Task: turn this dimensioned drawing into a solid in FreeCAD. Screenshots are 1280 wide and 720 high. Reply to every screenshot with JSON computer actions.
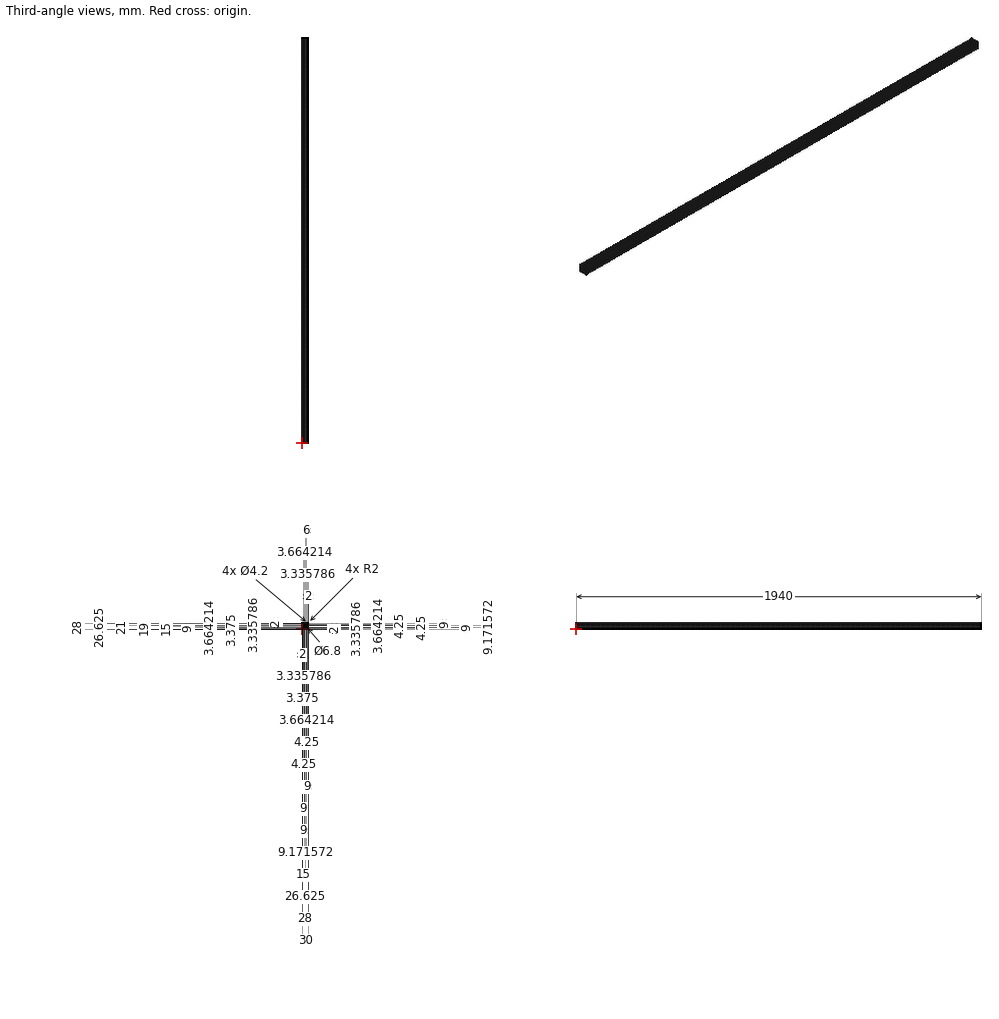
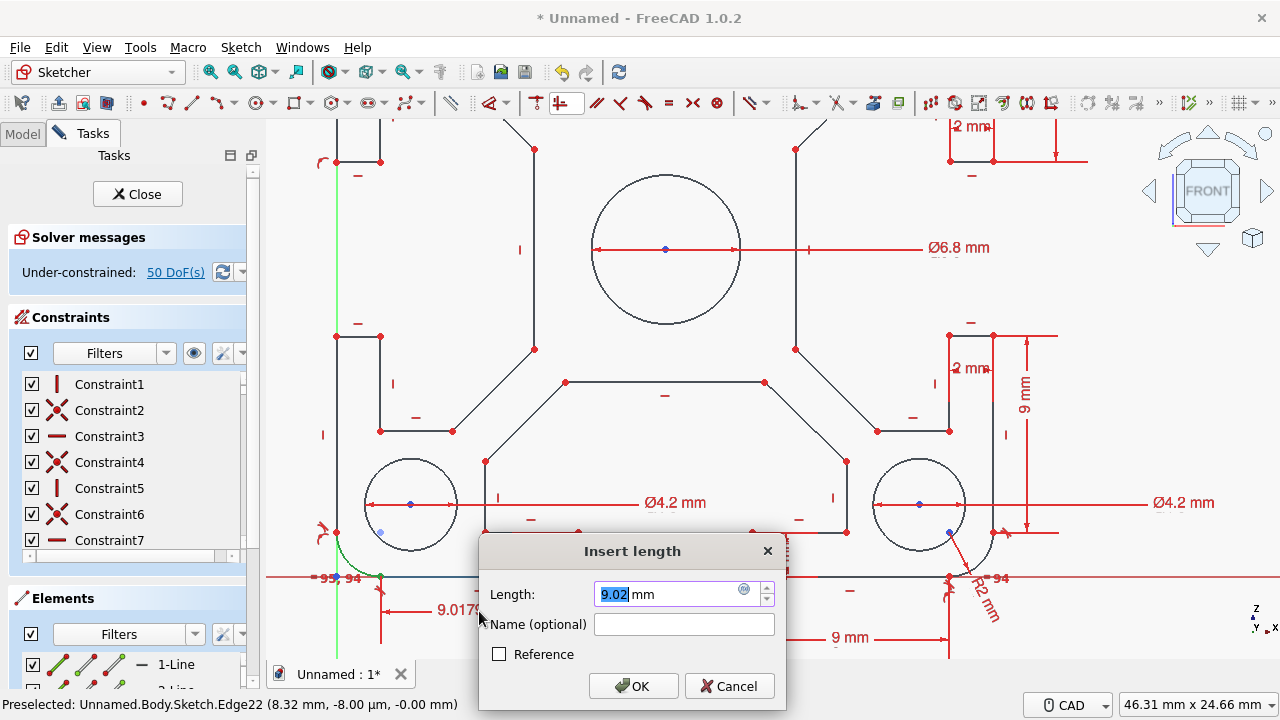
{"action": "type", "text": "9"}
{"action": "key", "text": "Return"}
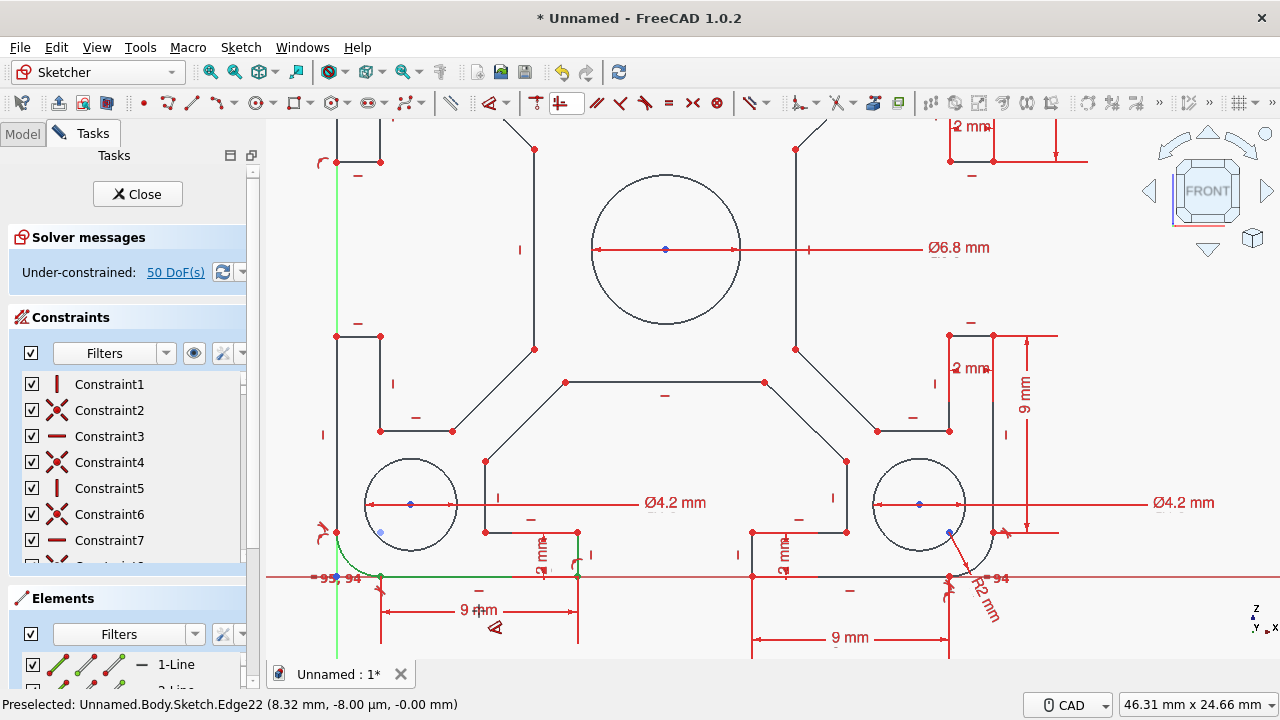
{"action": "left_click", "coordinate": [337, 474]}
{"action": "left_click", "coordinate": [303, 435]}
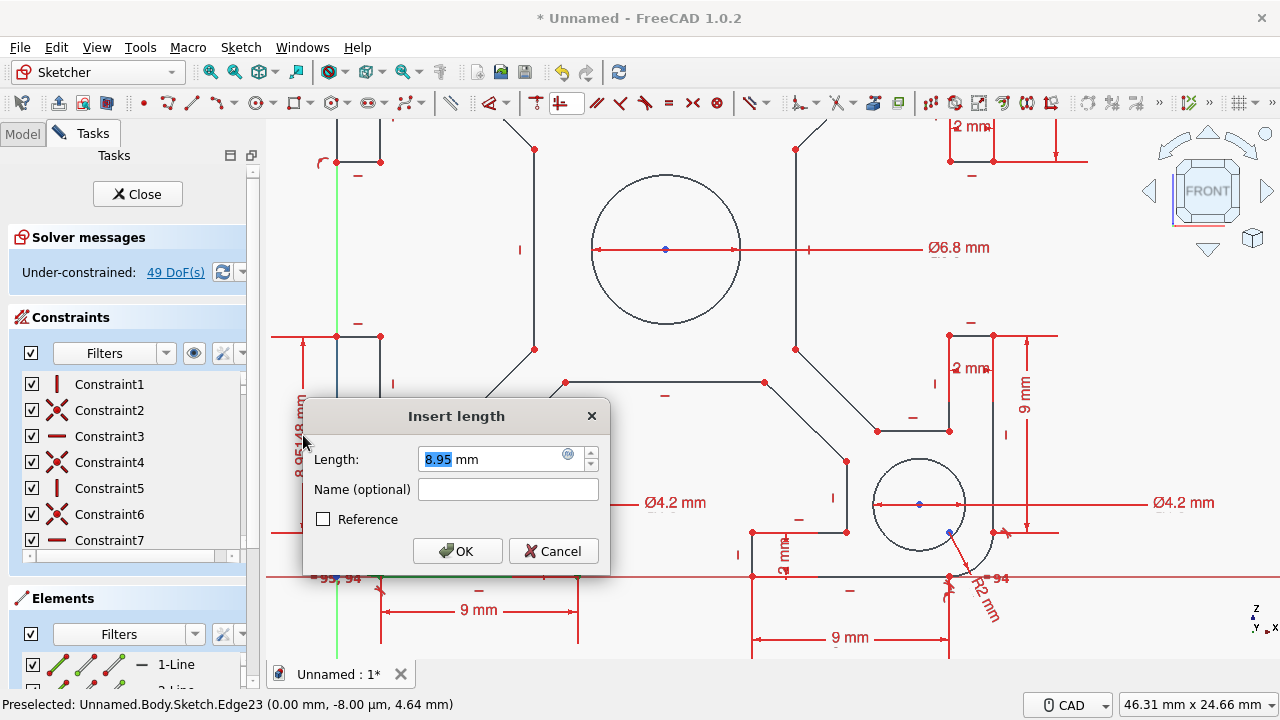
{"action": "type", "text": "9"}
{"action": "key", "text": "Return"}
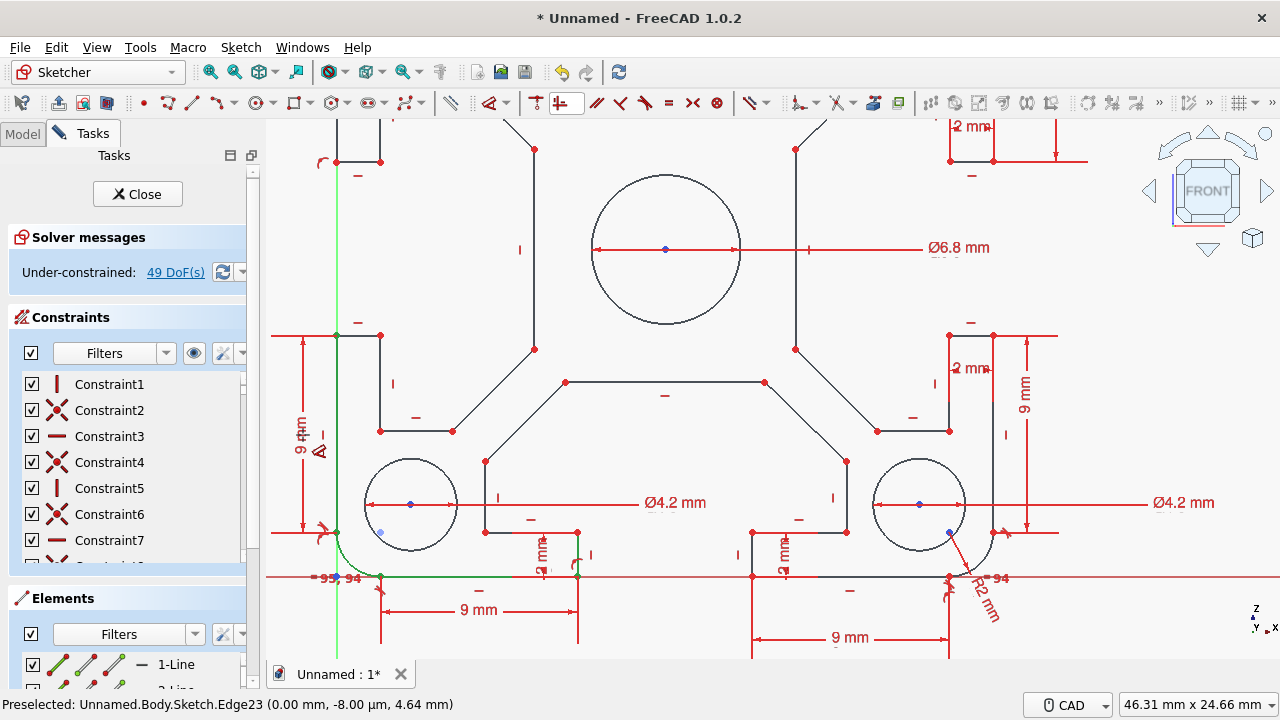
{"action": "left_click", "coordinate": [350, 336]}
{"action": "left_click", "coordinate": [358, 370]}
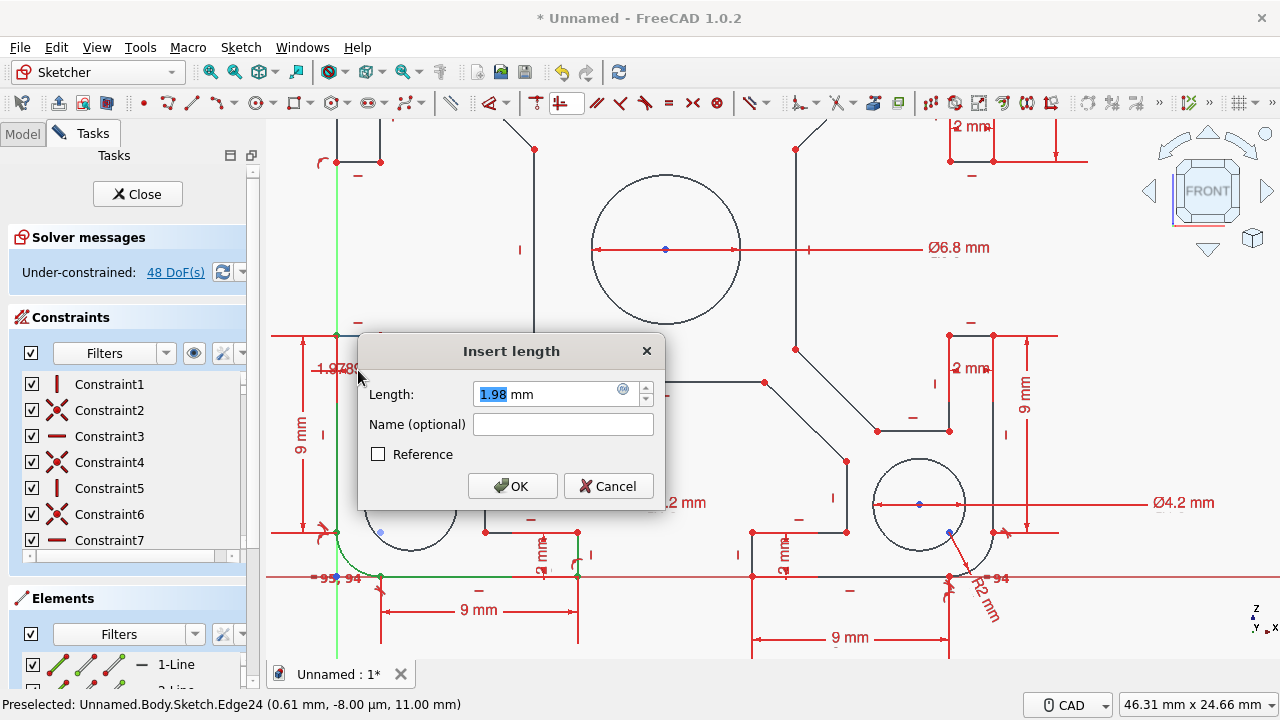
{"action": "type", "text": "2"}
{"action": "key", "text": "Return"}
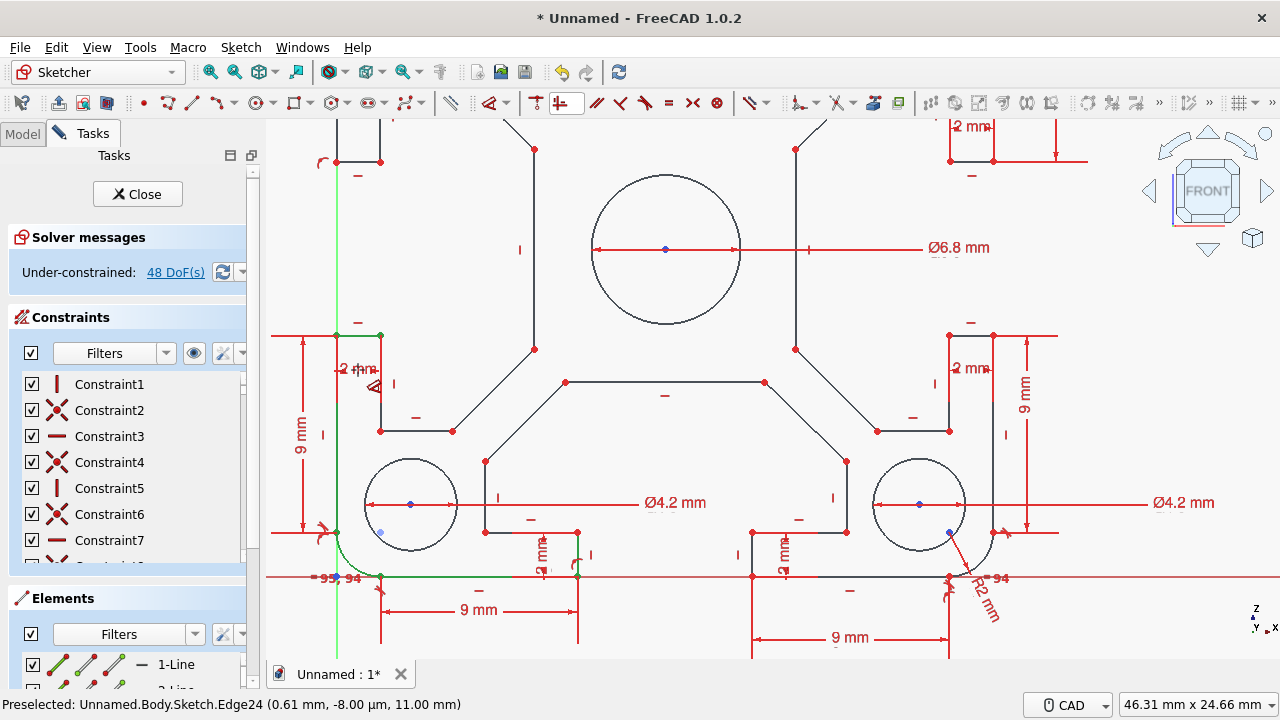
{"action": "left_click", "coordinate": [367, 162]}
{"action": "left_click", "coordinate": [358, 196]}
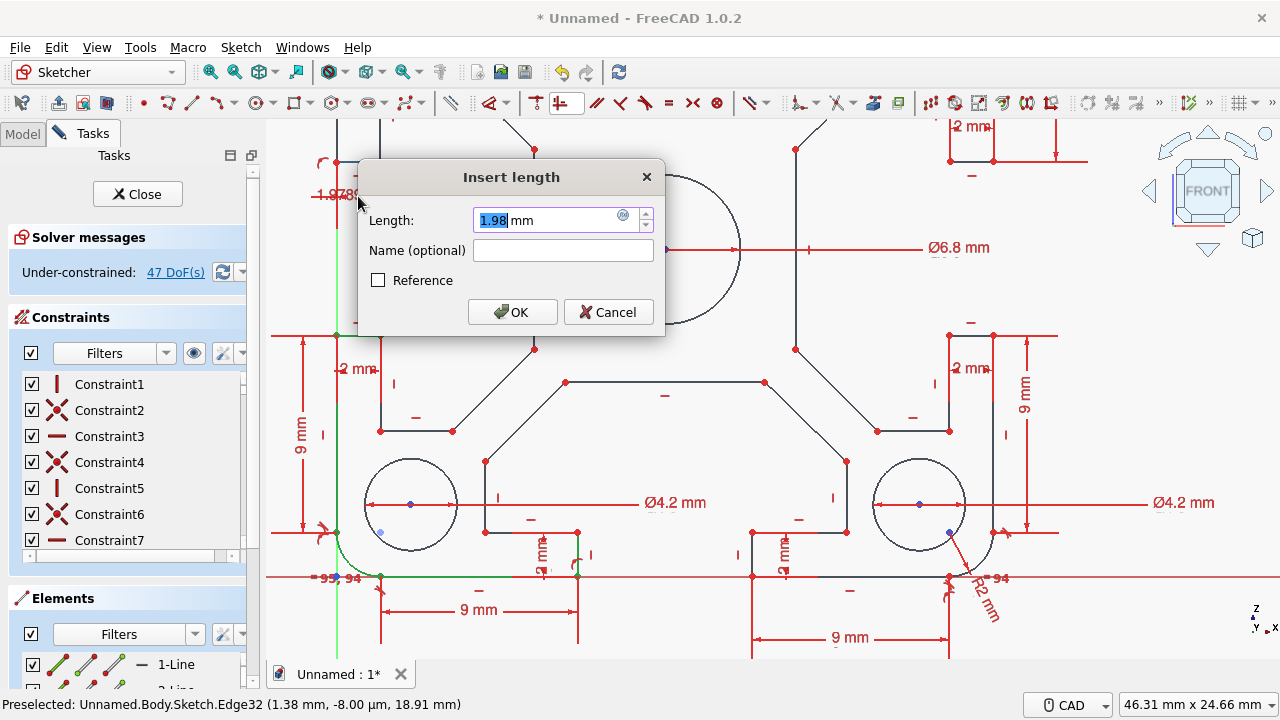
{"action": "type", "text": "2"}
{"action": "key", "text": "Return"}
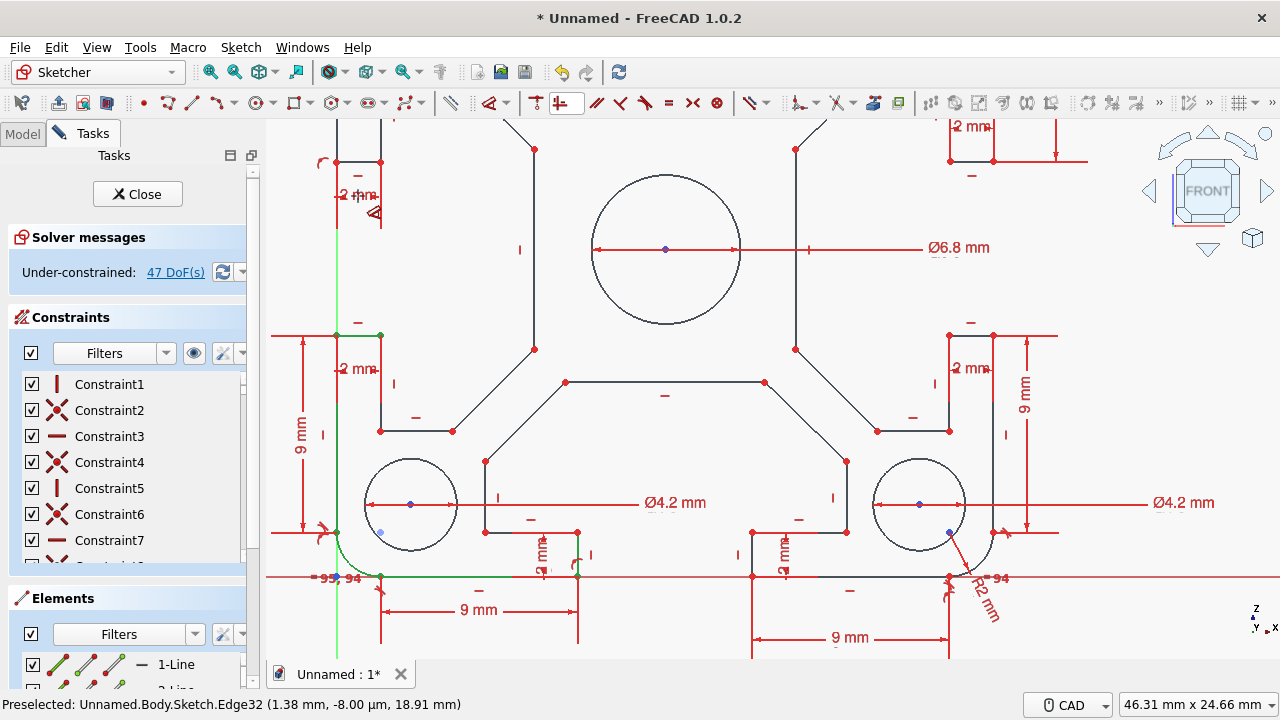
{"action": "scroll", "coordinate": [752, 560], "scroll_direction": "down", "scroll_amount": 3}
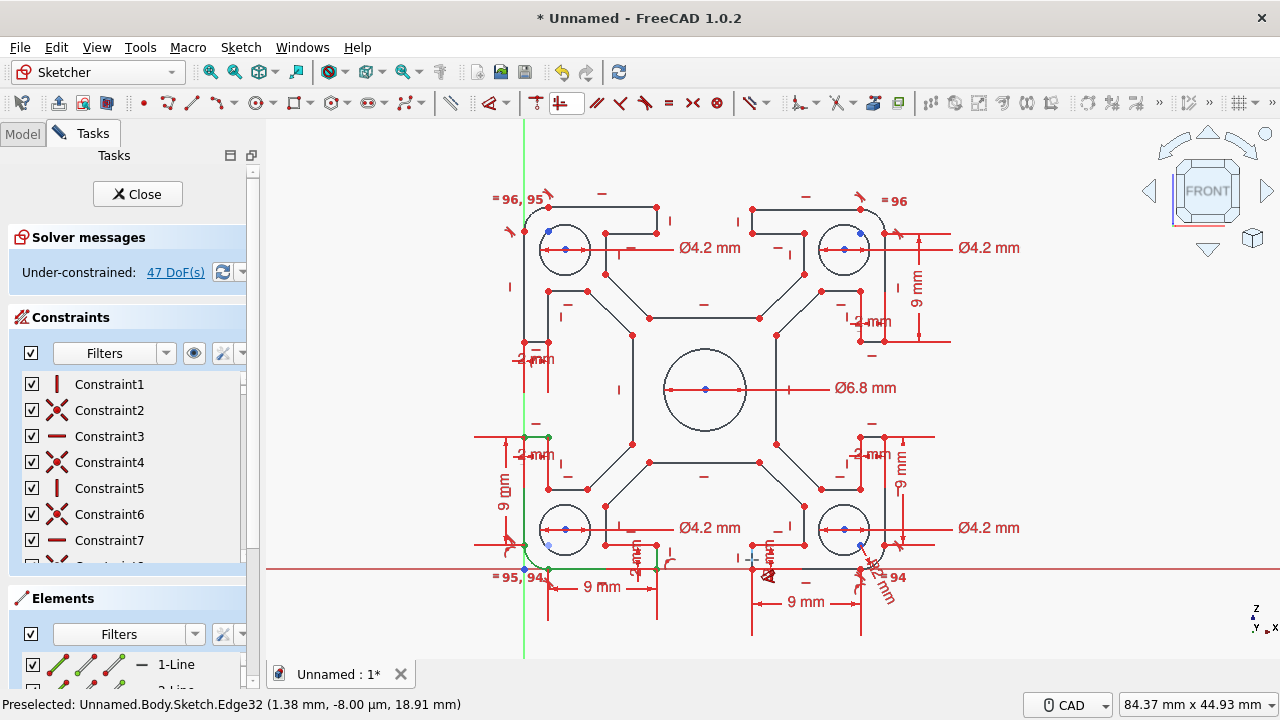
{"action": "left_click", "coordinate": [524, 309]}
{"action": "left_click", "coordinate": [490, 287]}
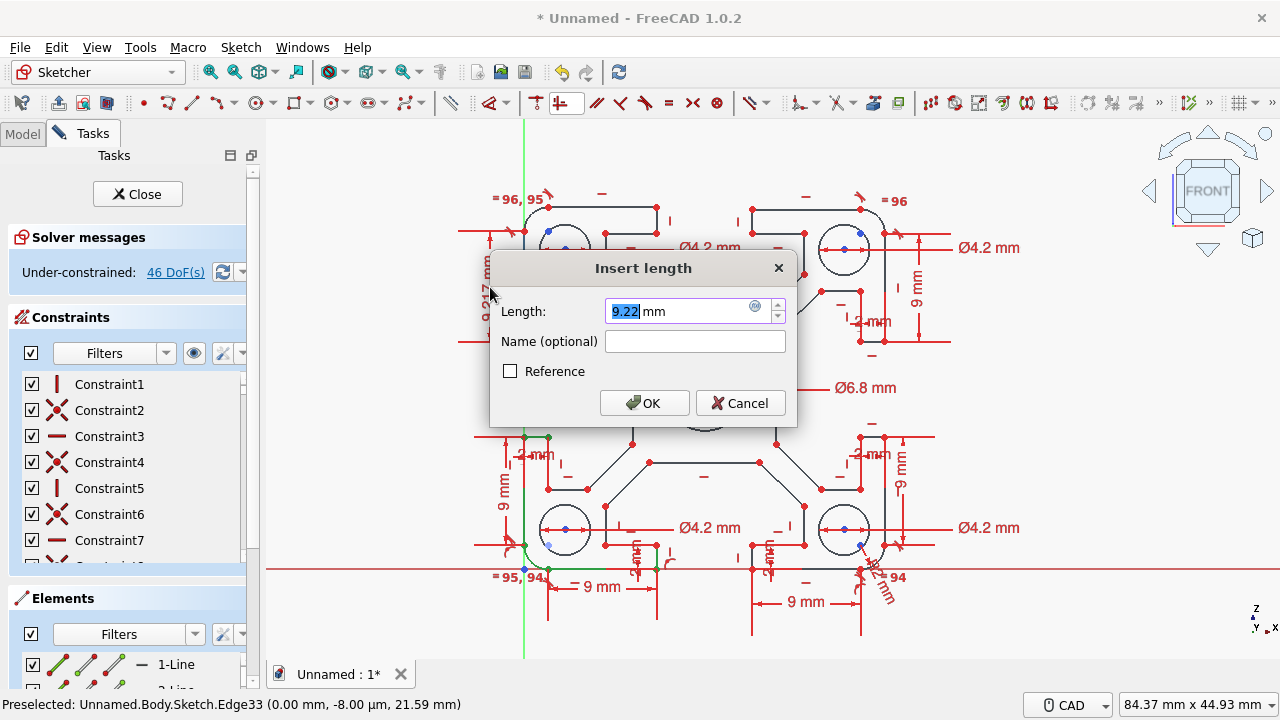
{"action": "type", "text": "9"}
{"action": "key", "text": "Return"}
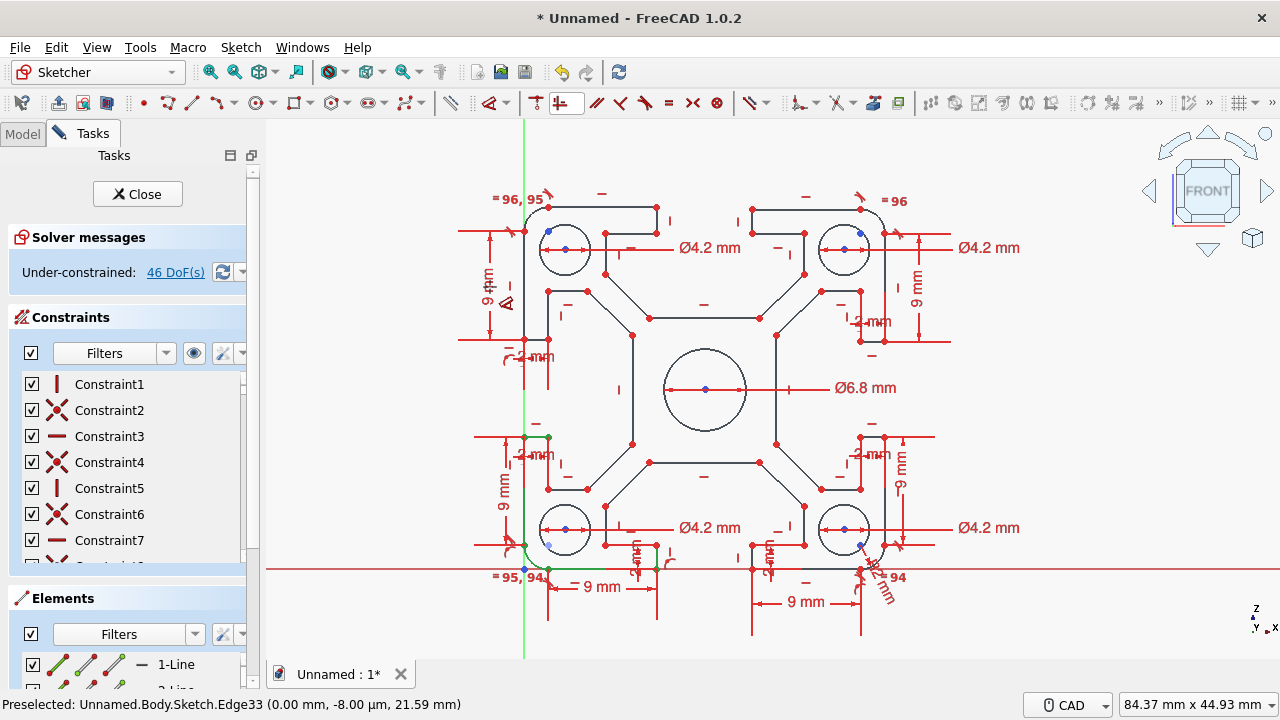
{"action": "left_click", "coordinate": [581, 207]}
{"action": "left_click", "coordinate": [603, 173]}